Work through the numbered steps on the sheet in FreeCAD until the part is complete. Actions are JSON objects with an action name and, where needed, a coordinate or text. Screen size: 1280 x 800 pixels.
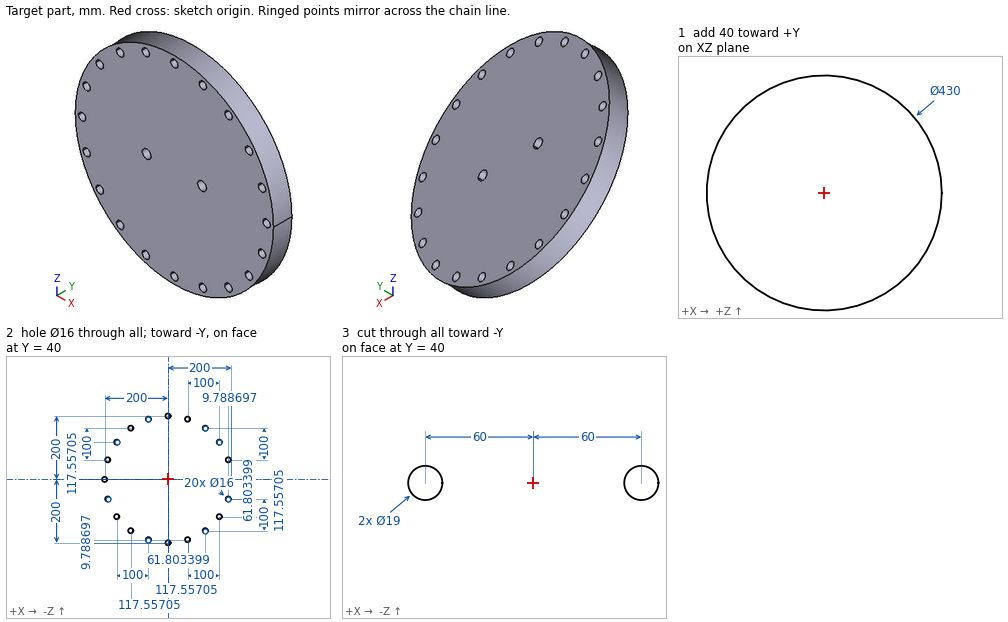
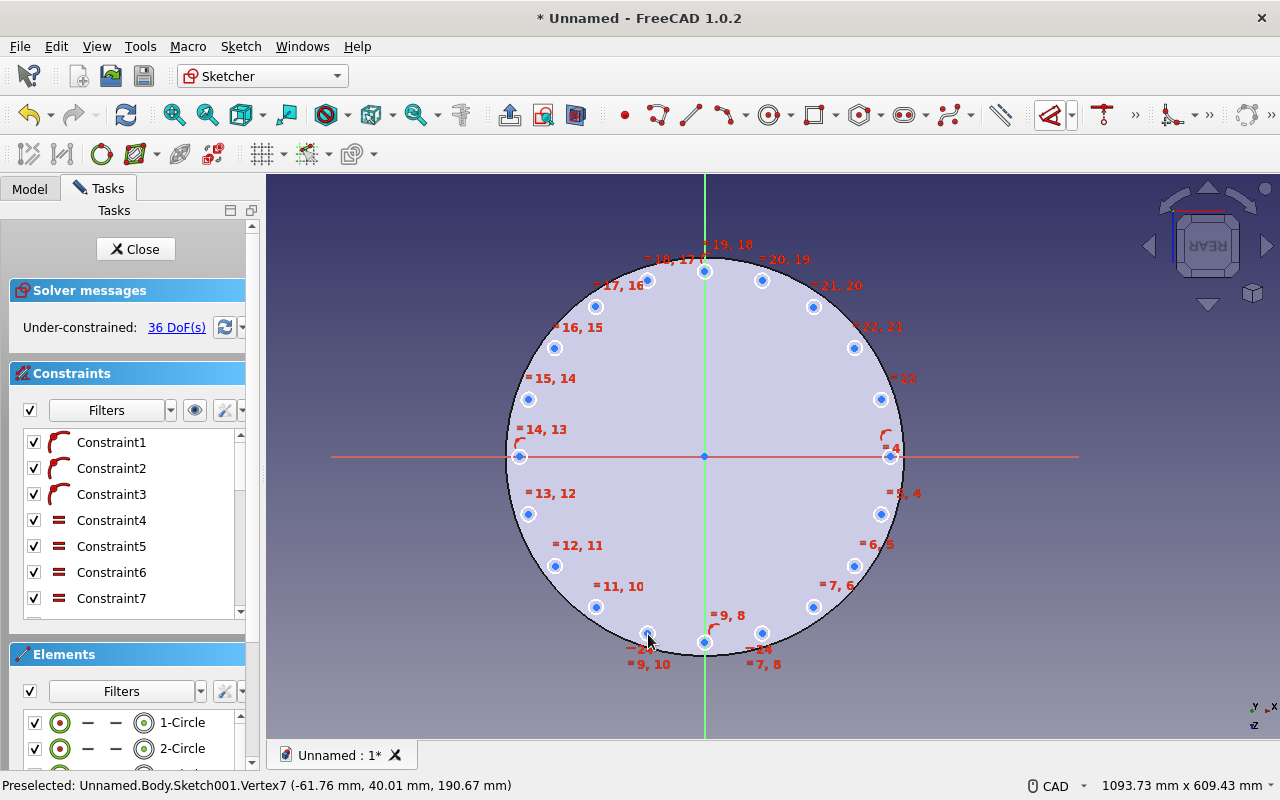
{"action": "left_click", "coordinate": [814, 607]}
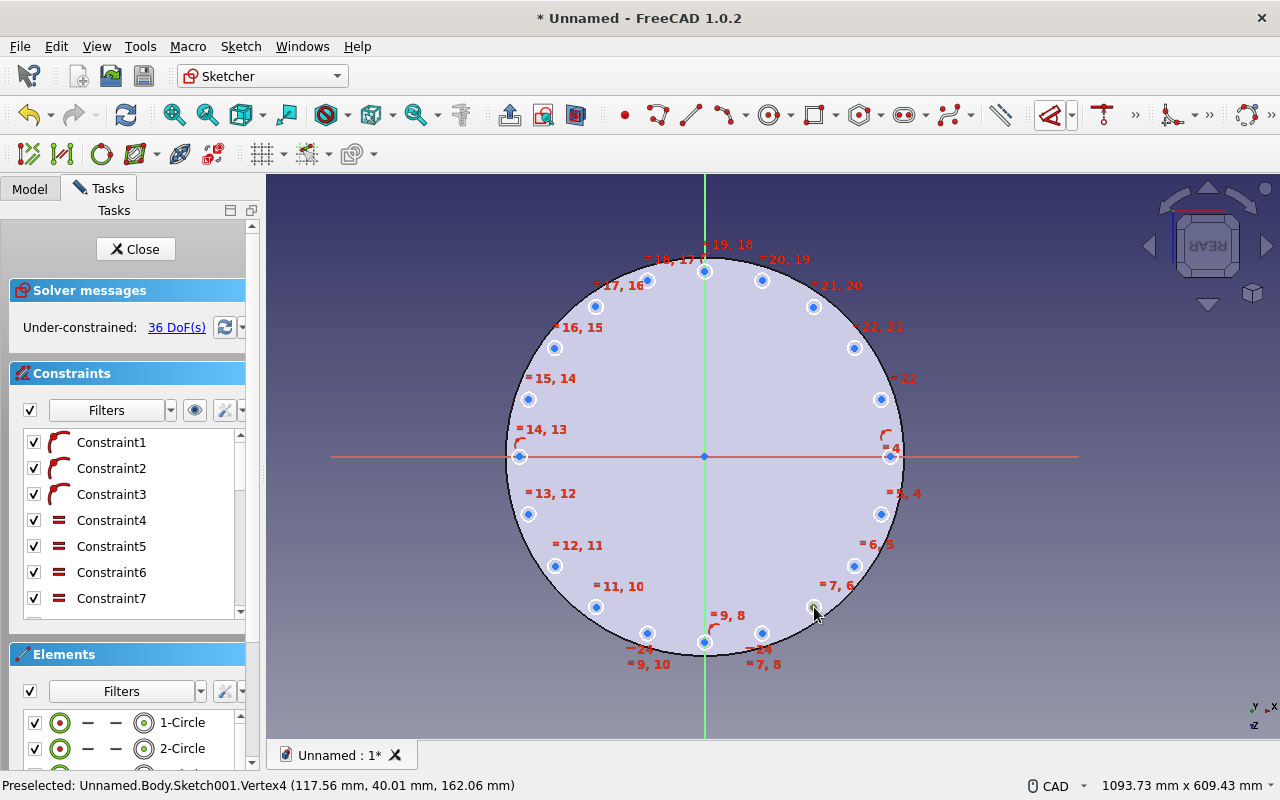
{"action": "left_click", "coordinate": [596, 607]}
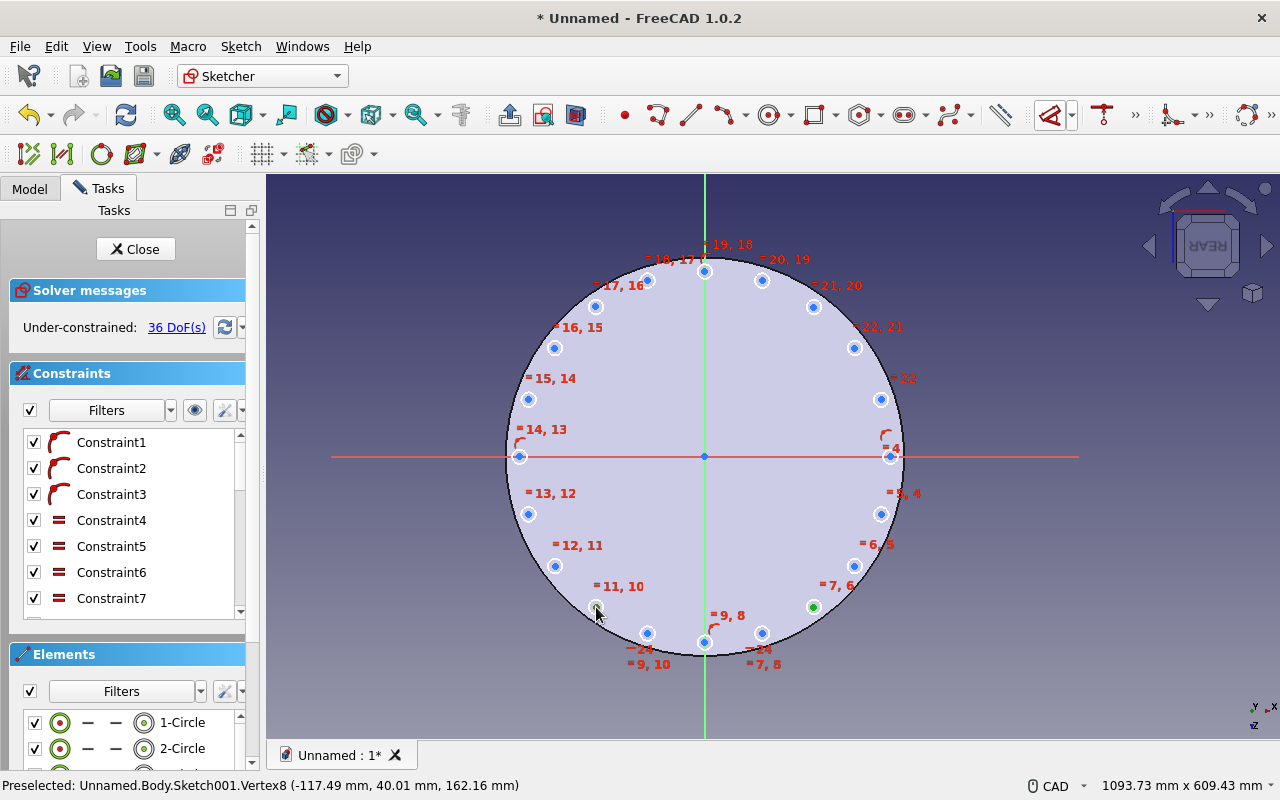
{"action": "key", "text": "h"}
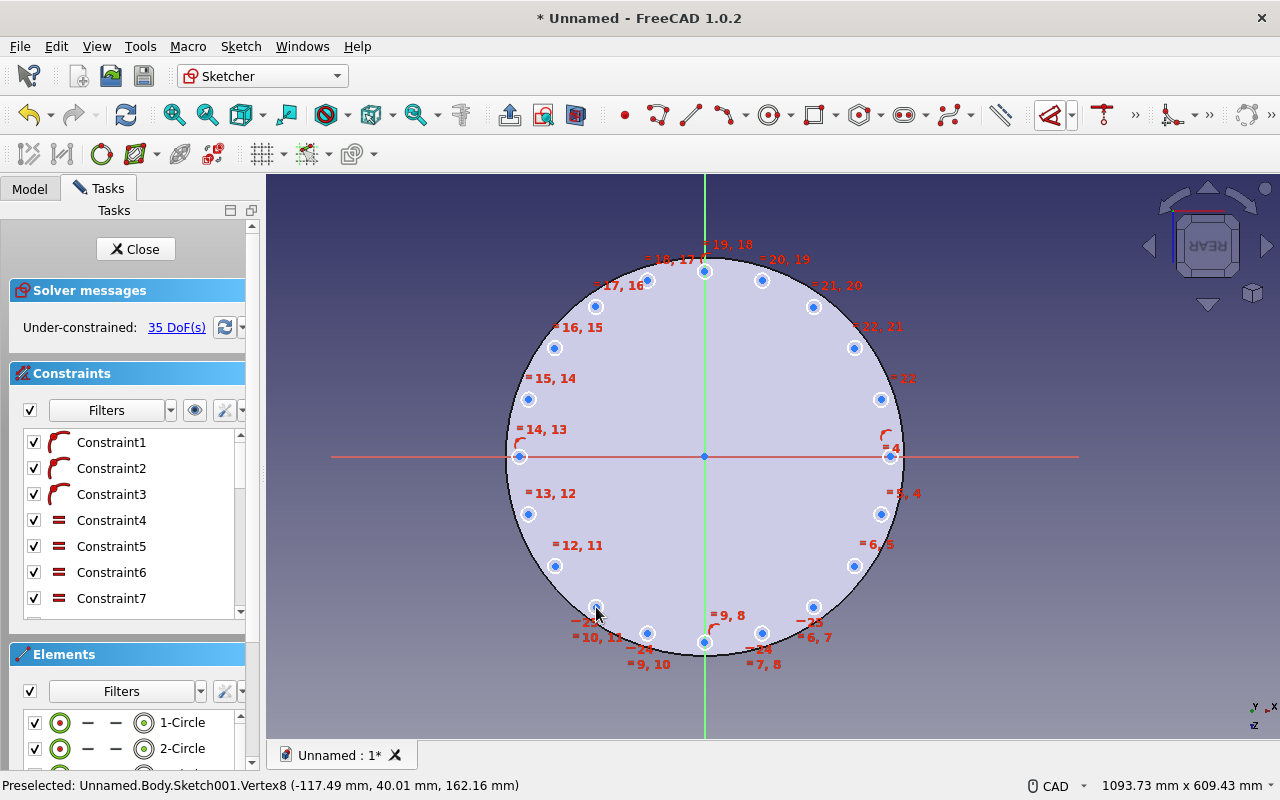
{"action": "left_click", "coordinate": [855, 566]}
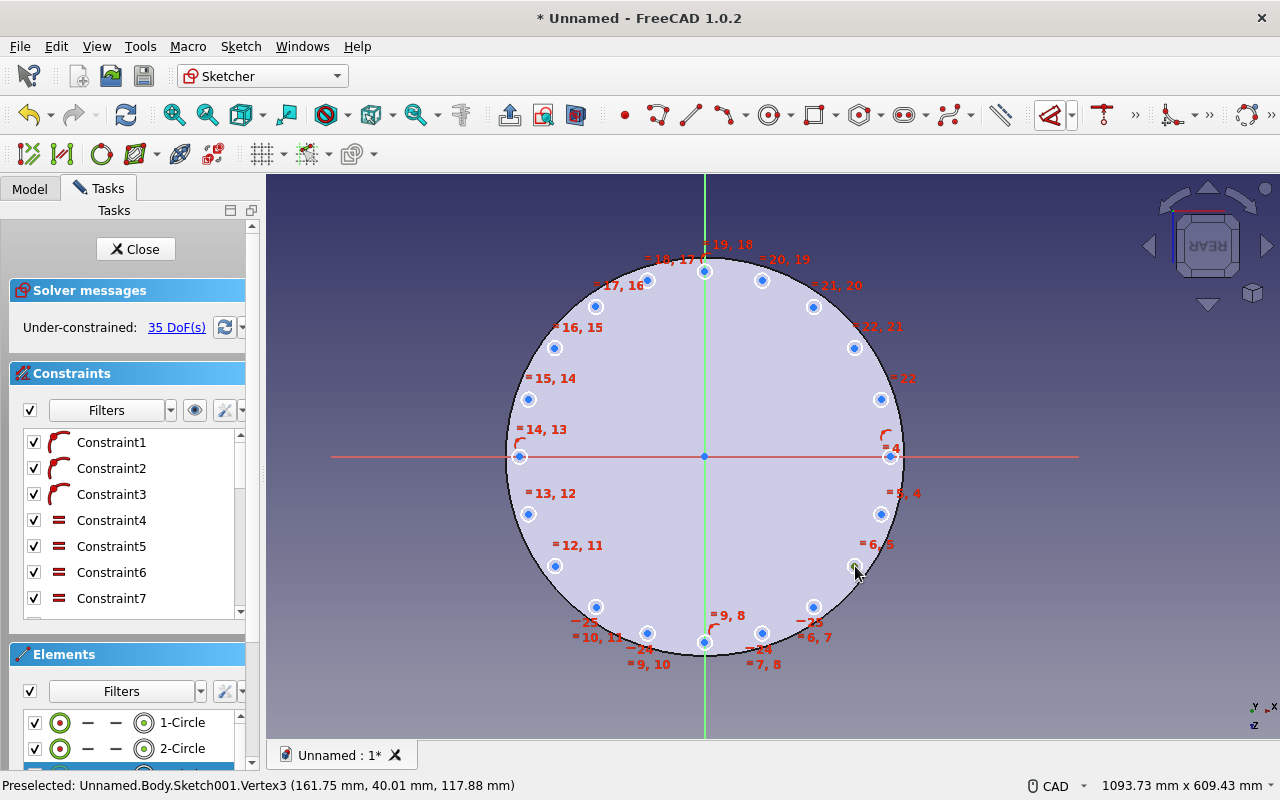
{"action": "left_click", "coordinate": [555, 566]}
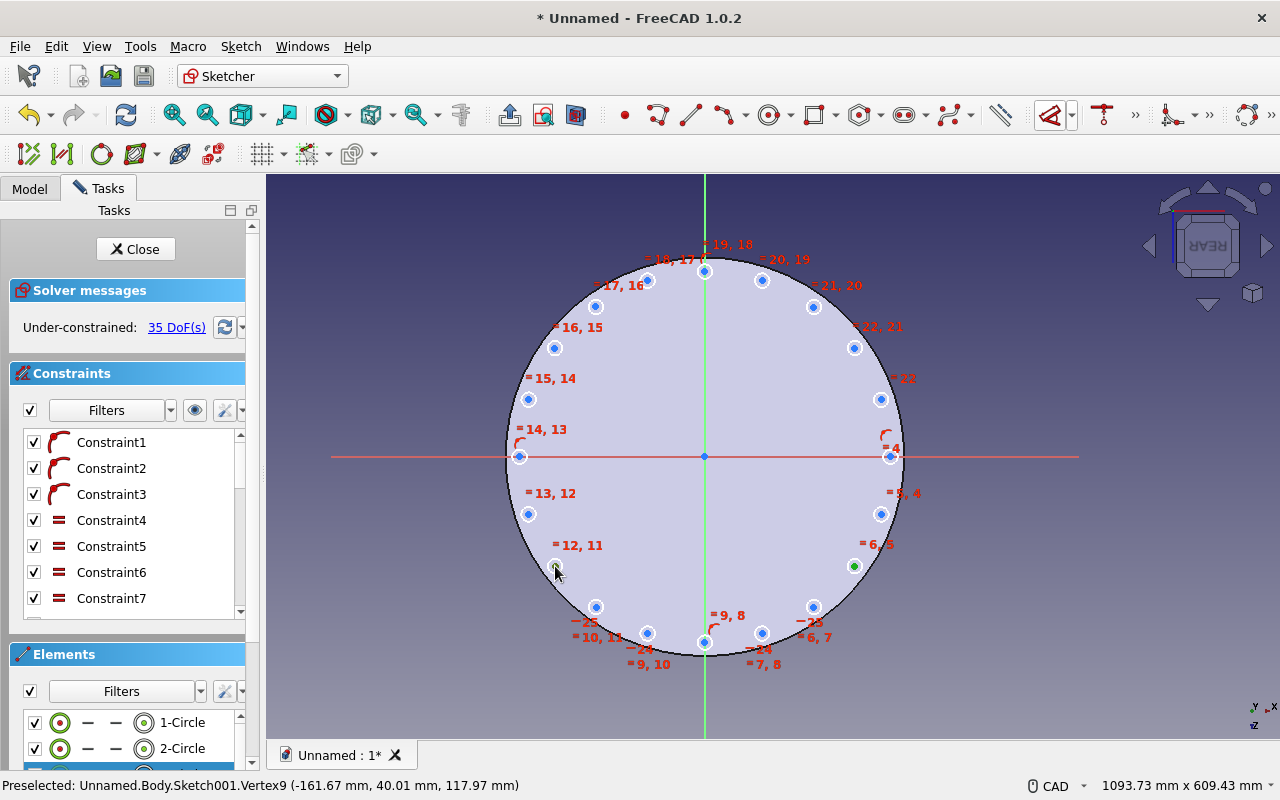
{"action": "key", "text": "h"}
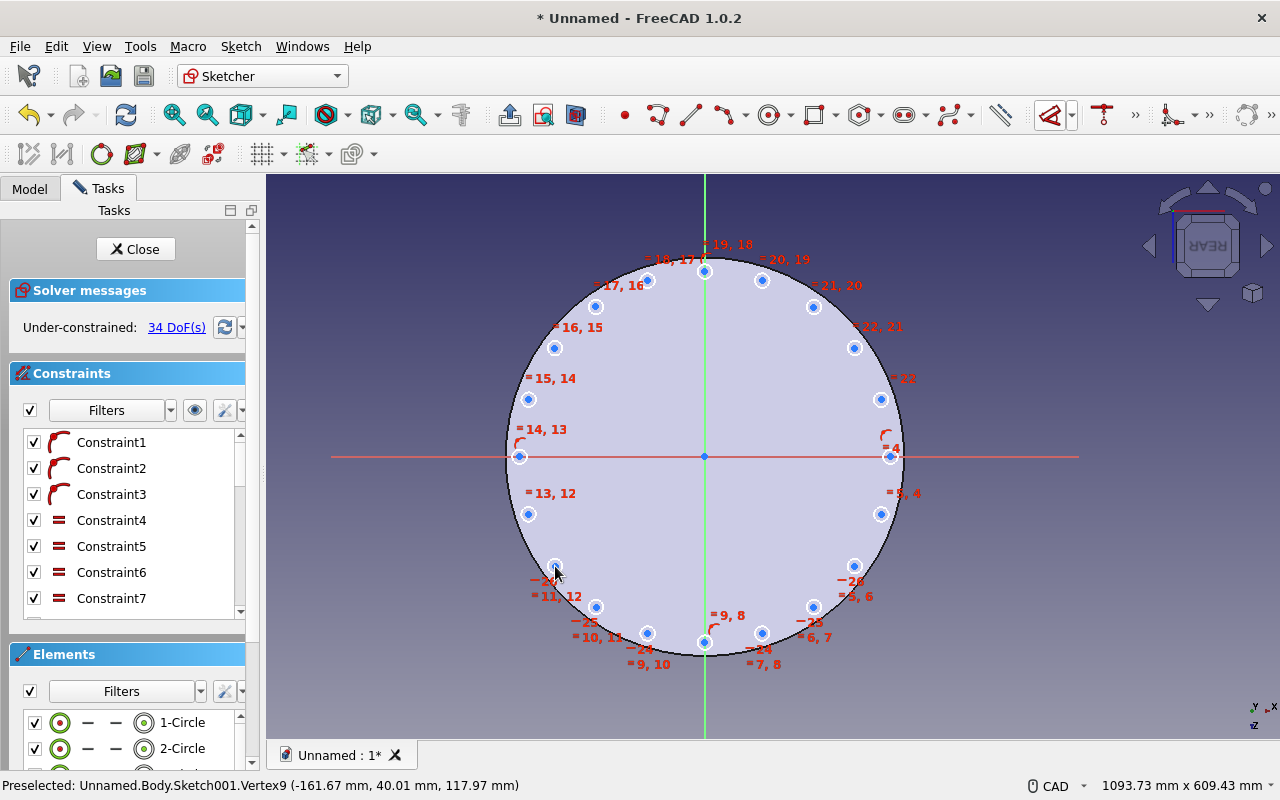
{"action": "left_click", "coordinate": [529, 514]}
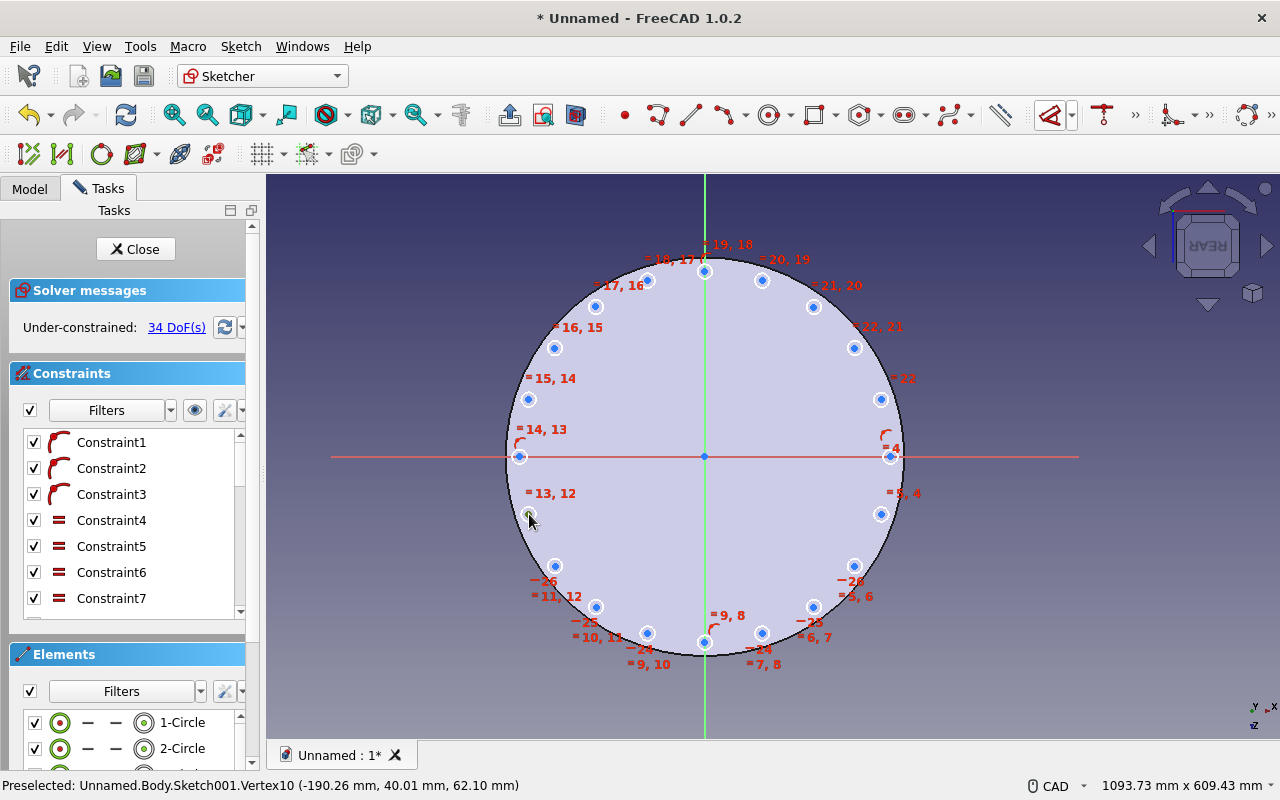
{"action": "left_click", "coordinate": [529, 400]}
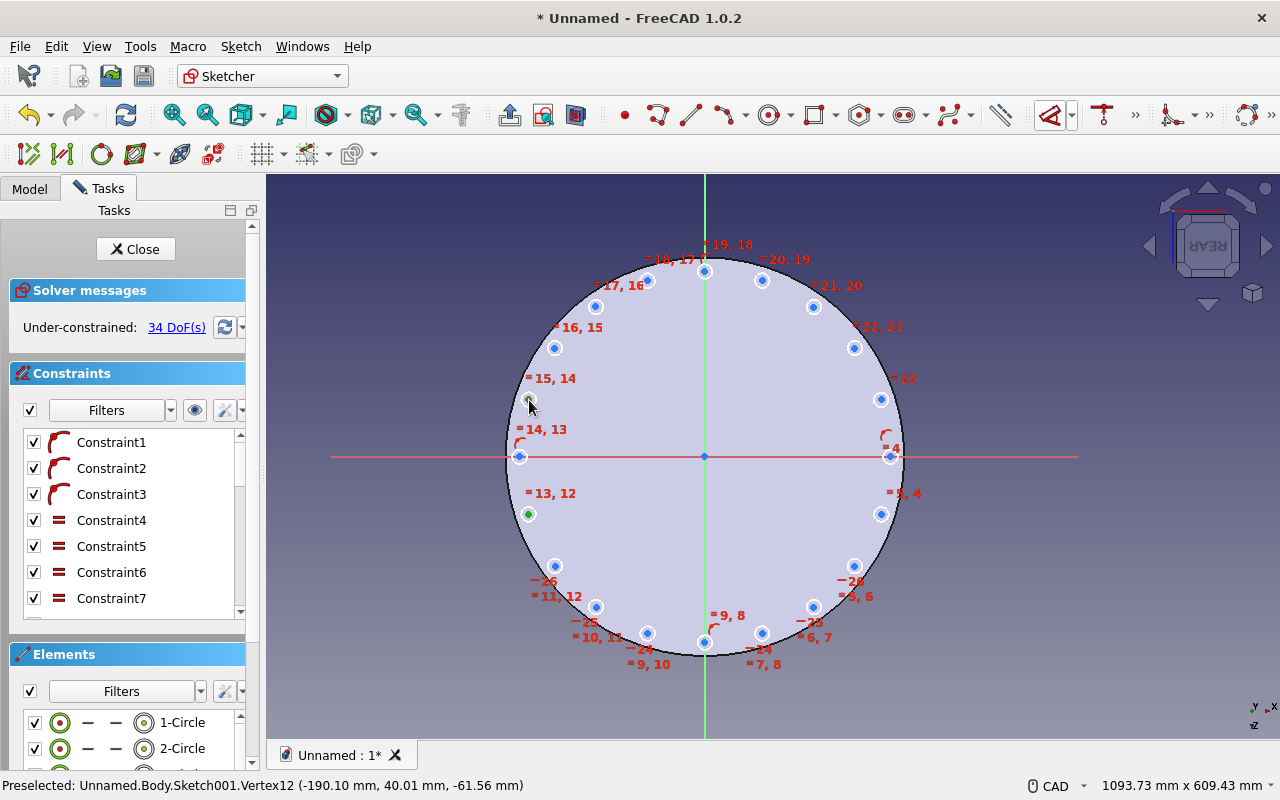
{"action": "key", "text": "v"}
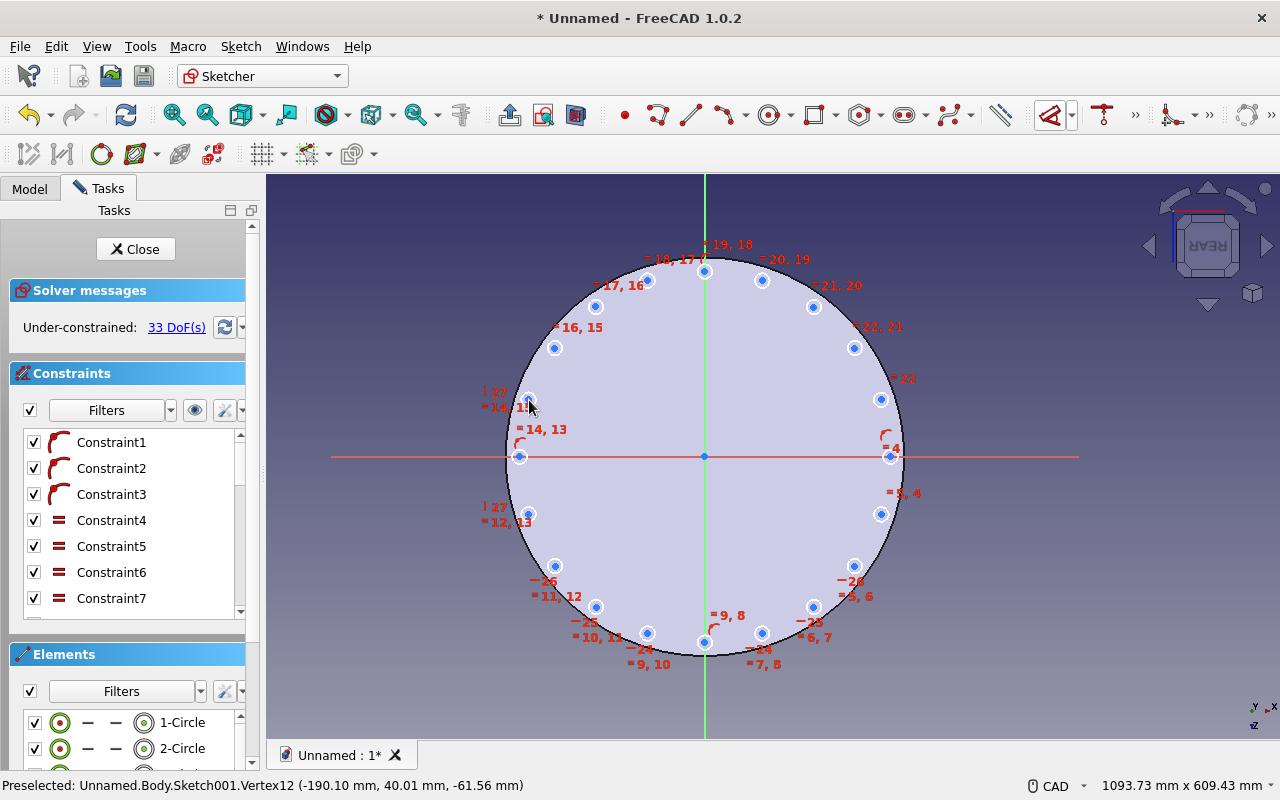
{"action": "left_click", "coordinate": [555, 566]}